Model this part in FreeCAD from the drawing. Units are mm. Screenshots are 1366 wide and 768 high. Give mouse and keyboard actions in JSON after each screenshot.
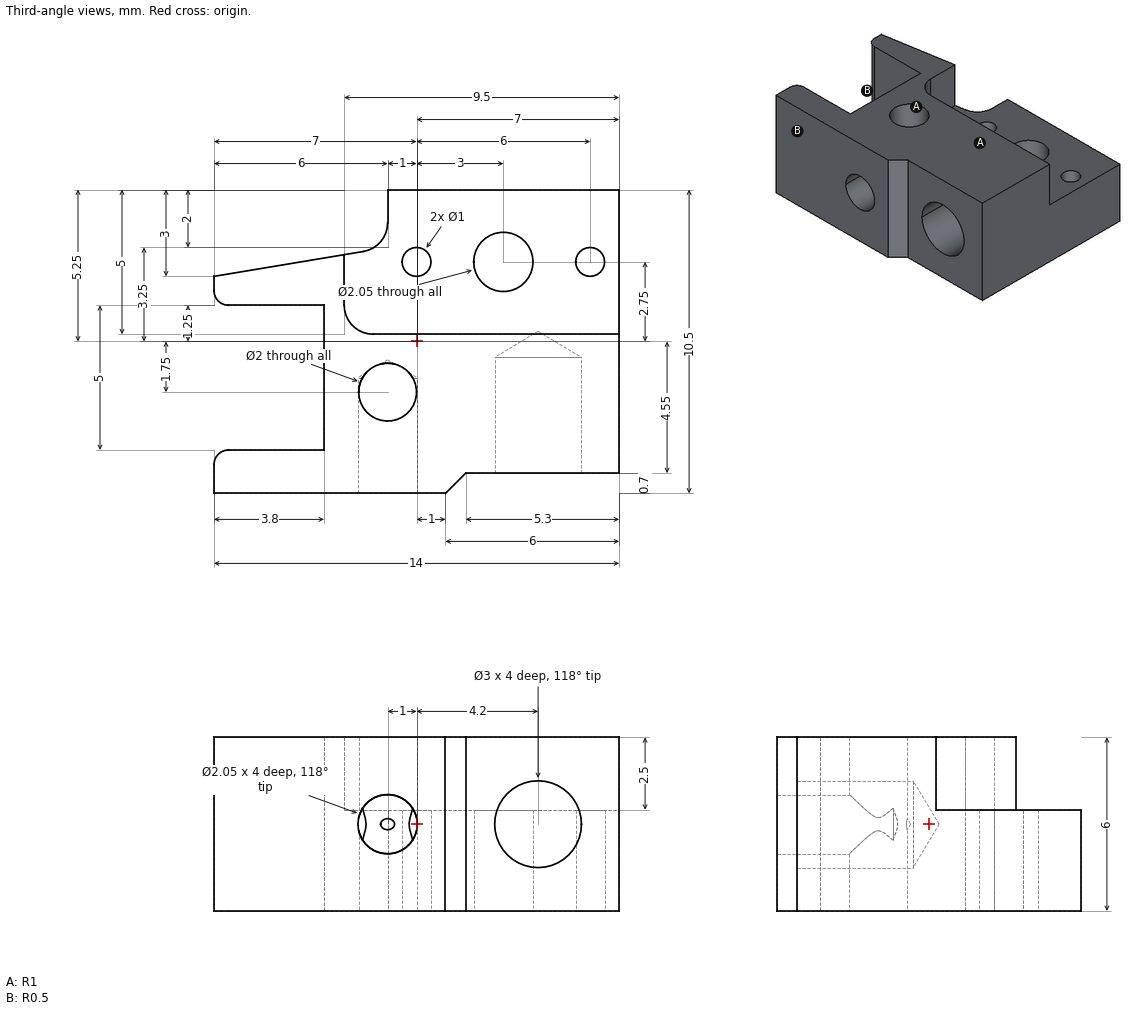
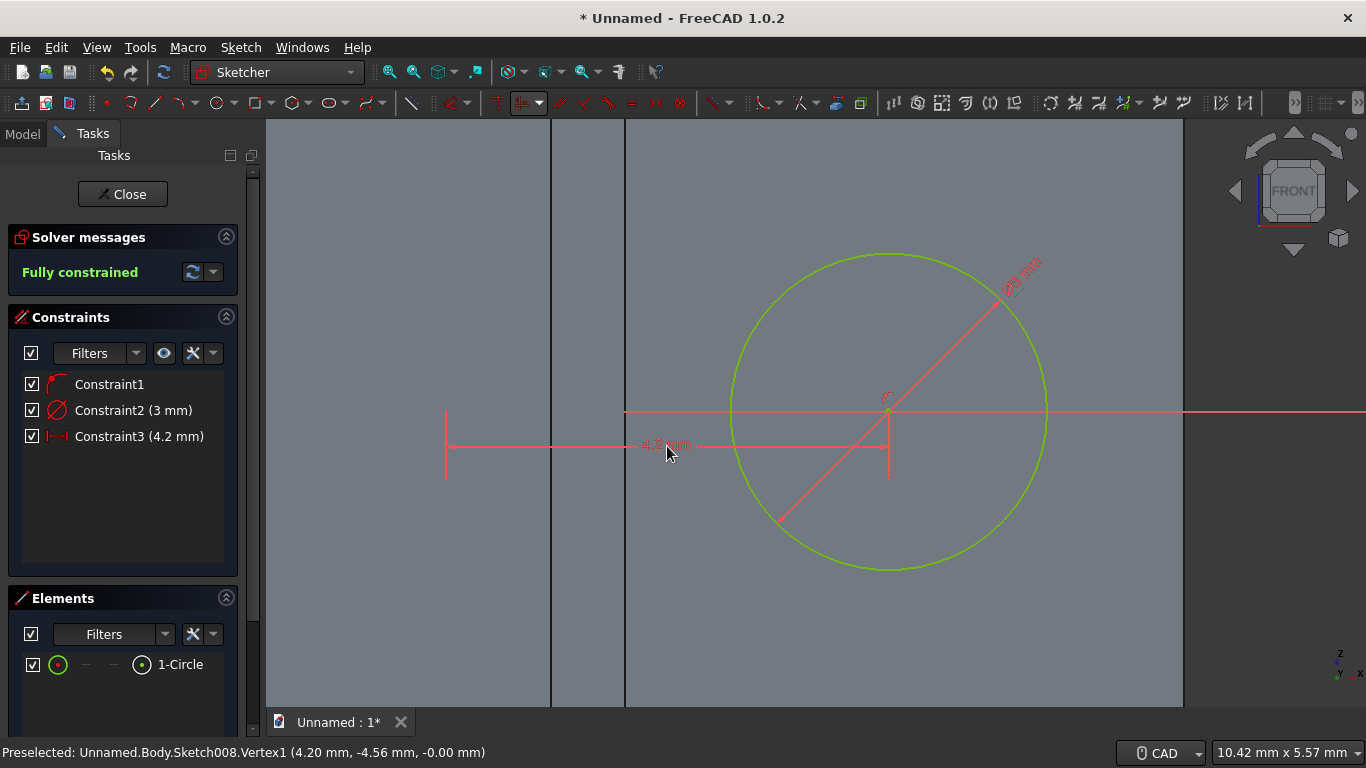
{"action": "left_click", "coordinate": [123, 194]}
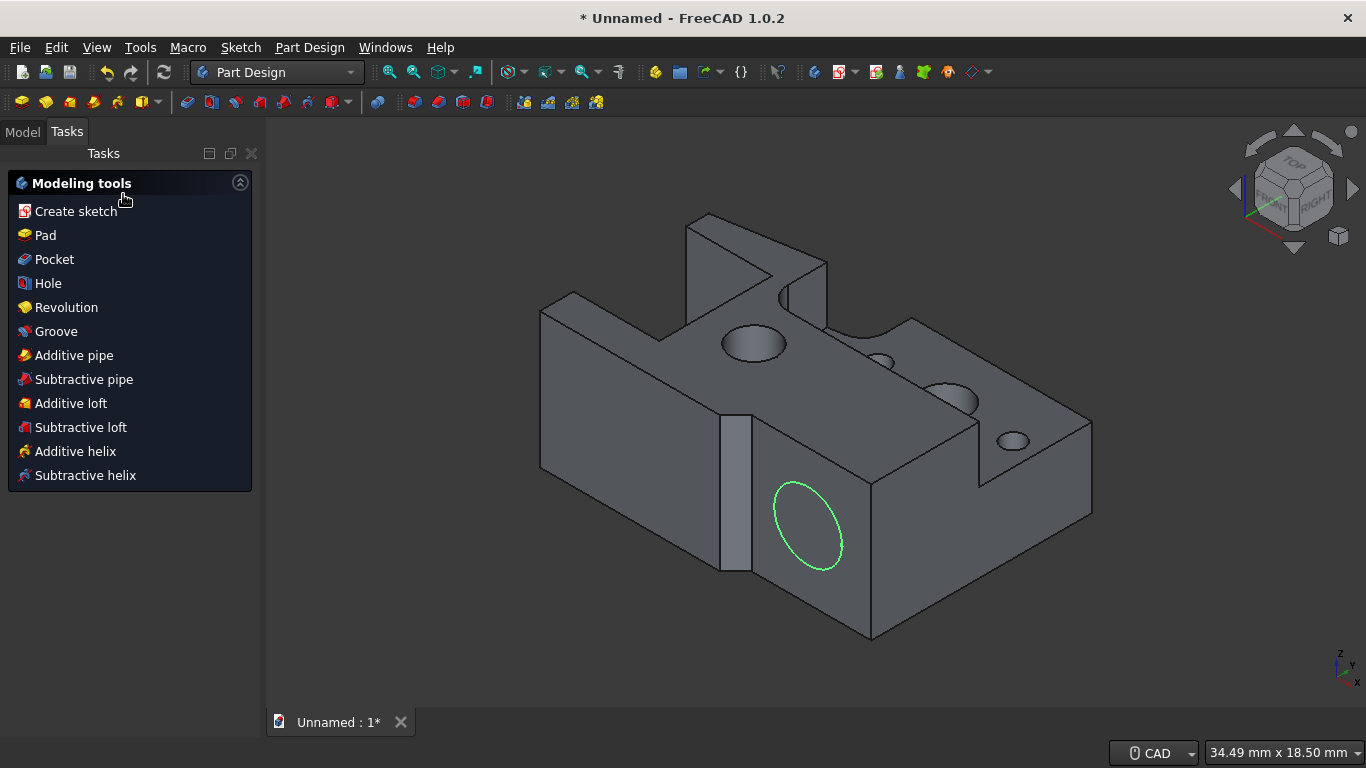
{"action": "left_click", "coordinate": [212, 102]}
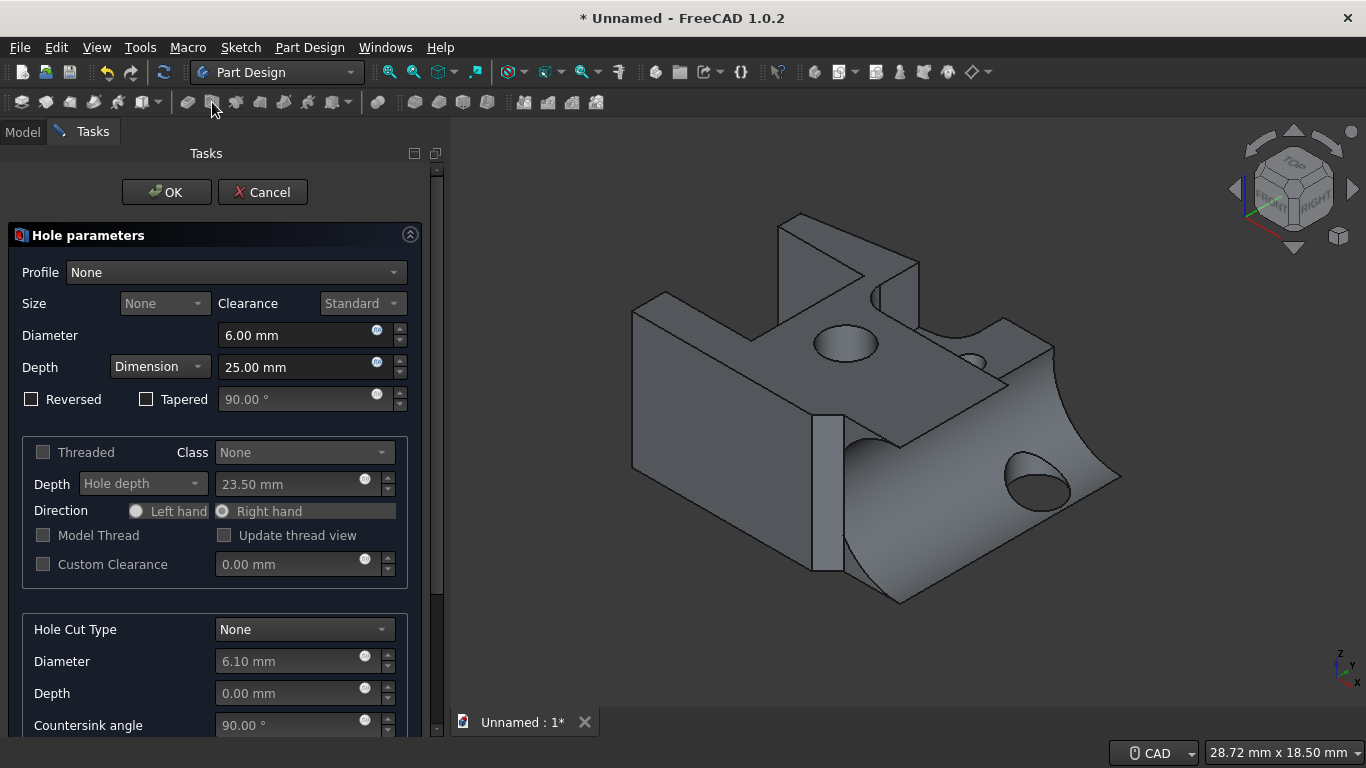
{"action": "triple_click", "coordinate": [305, 335]}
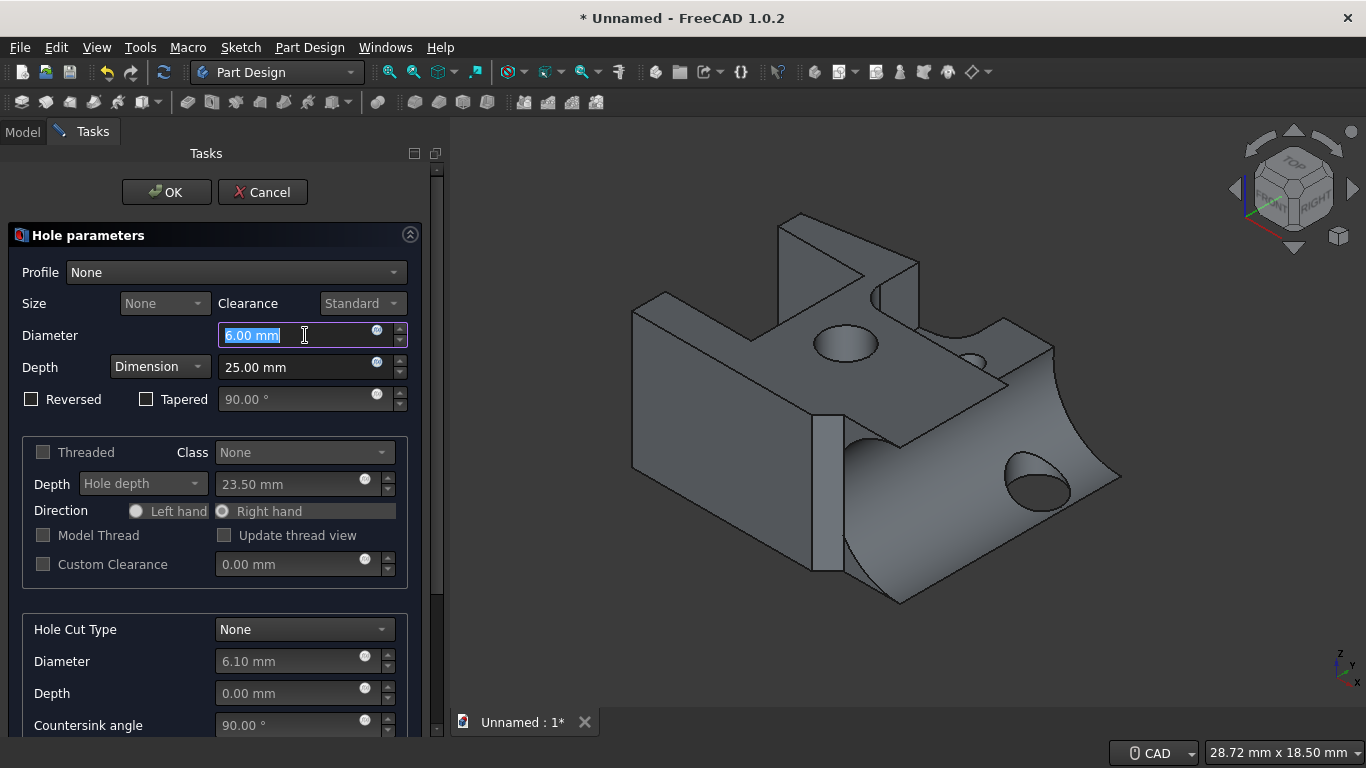
{"action": "type", "text": "3"}
{"action": "key", "text": "Tab"}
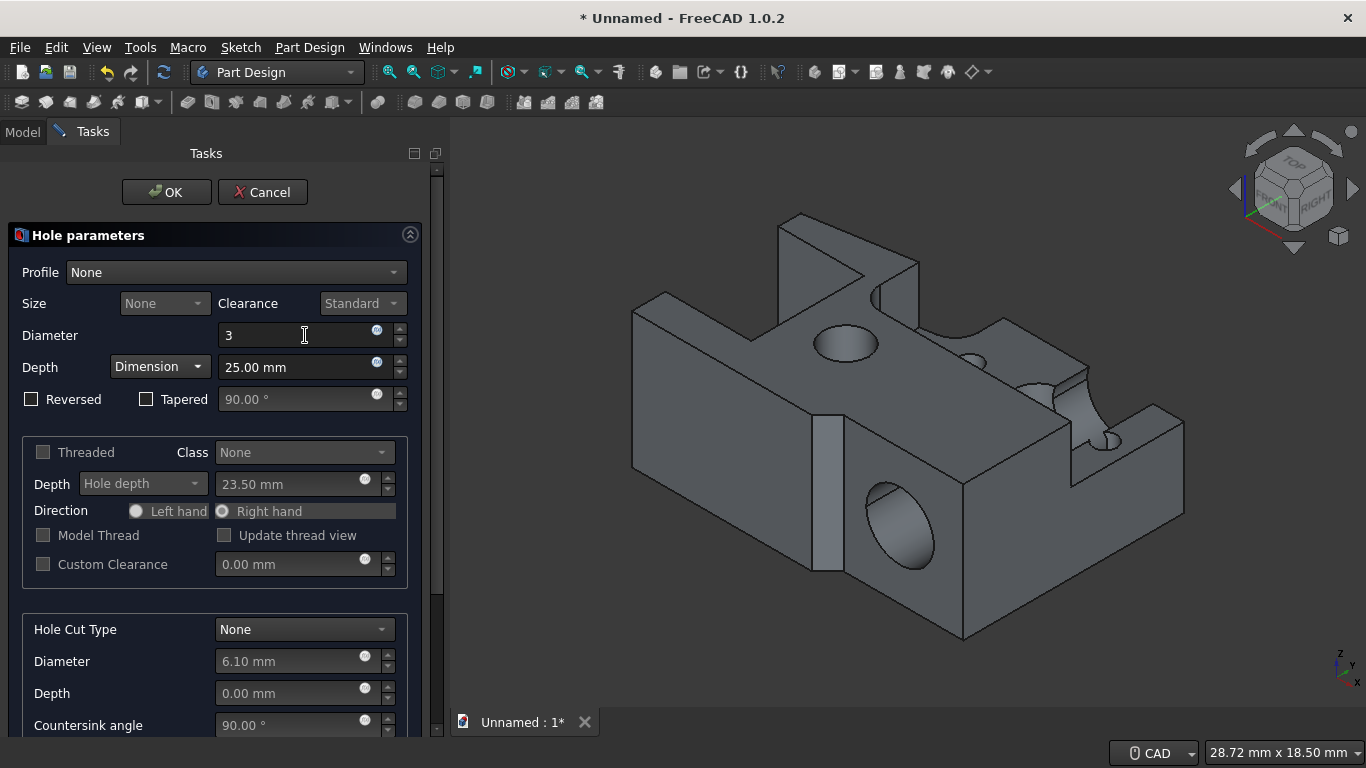
{"action": "triple_click", "coordinate": [305, 367]}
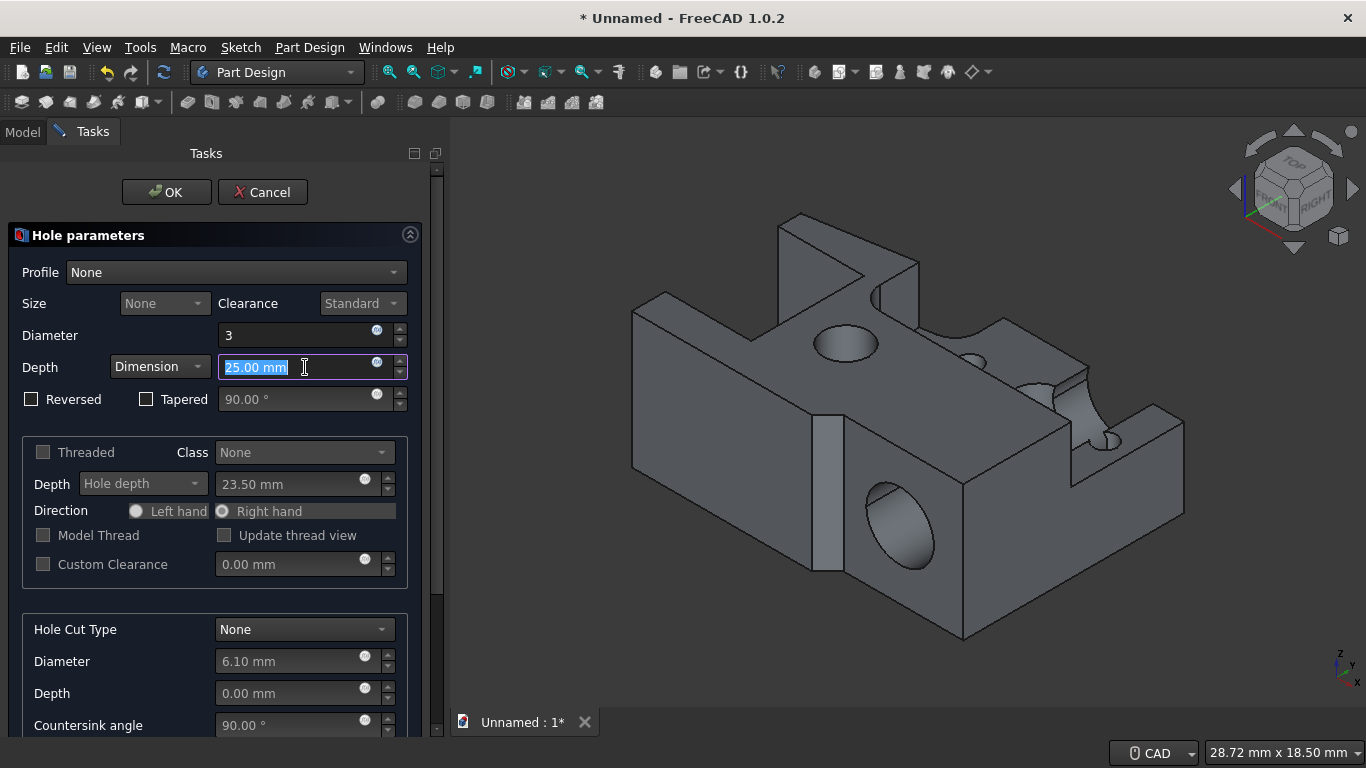
{"action": "type", "text": "4"}
{"action": "key", "text": "Tab"}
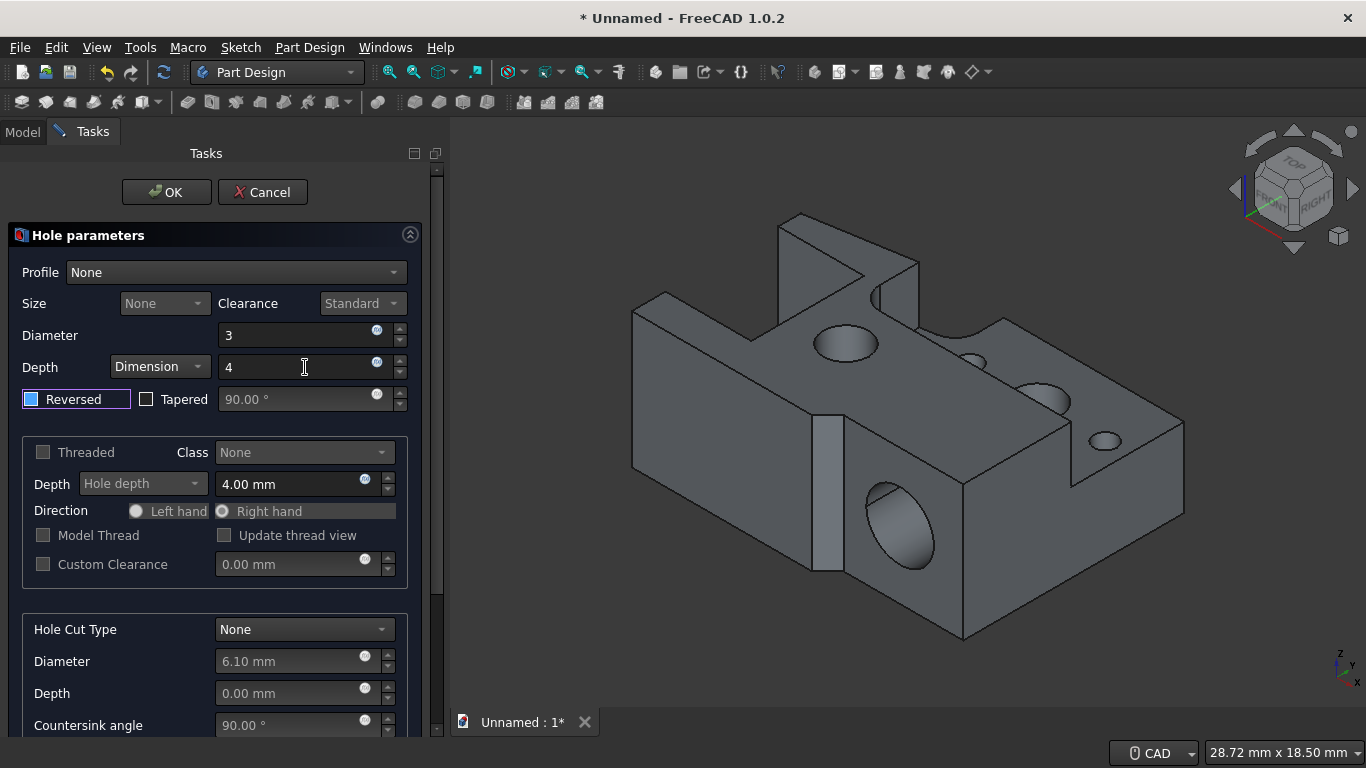
{"action": "left_click", "coordinate": [167, 192]}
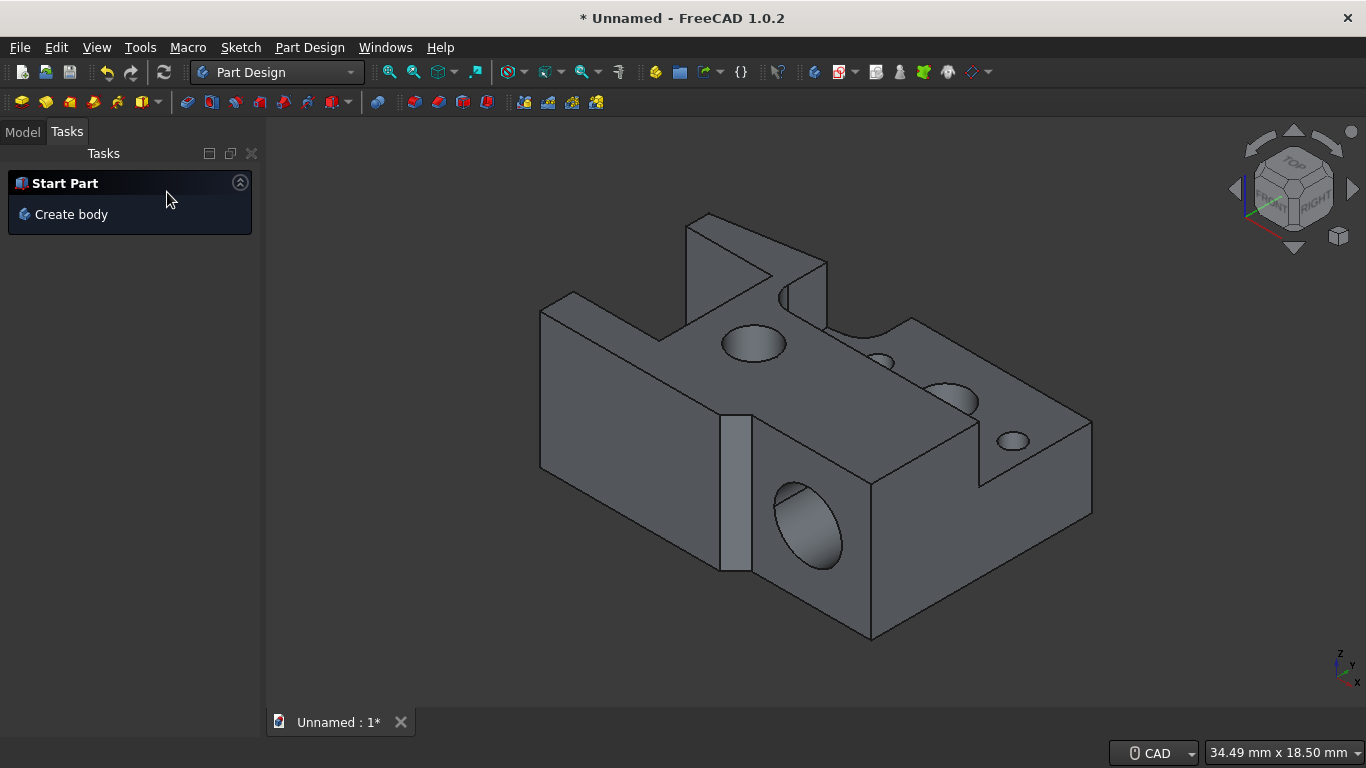
{"action": "key", "text": "2"}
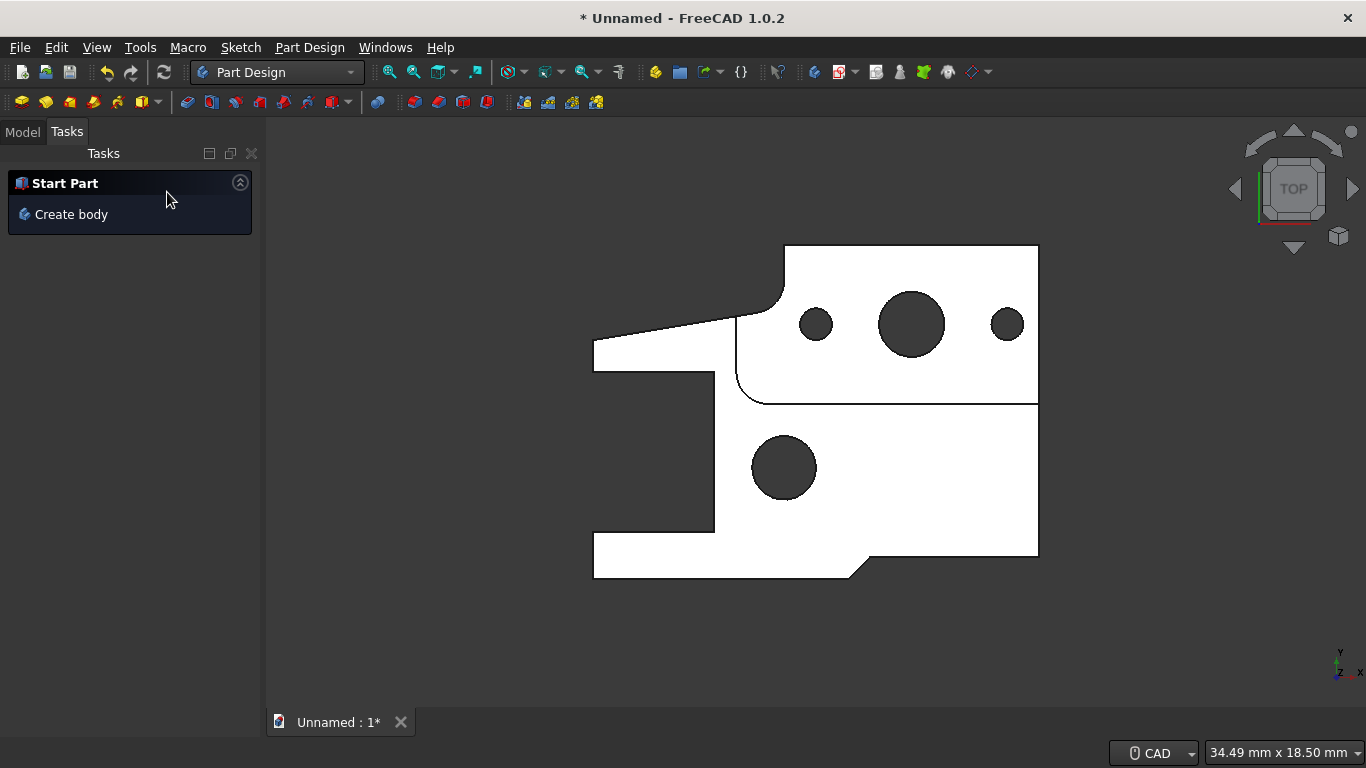
{"action": "key", "text": "0"}